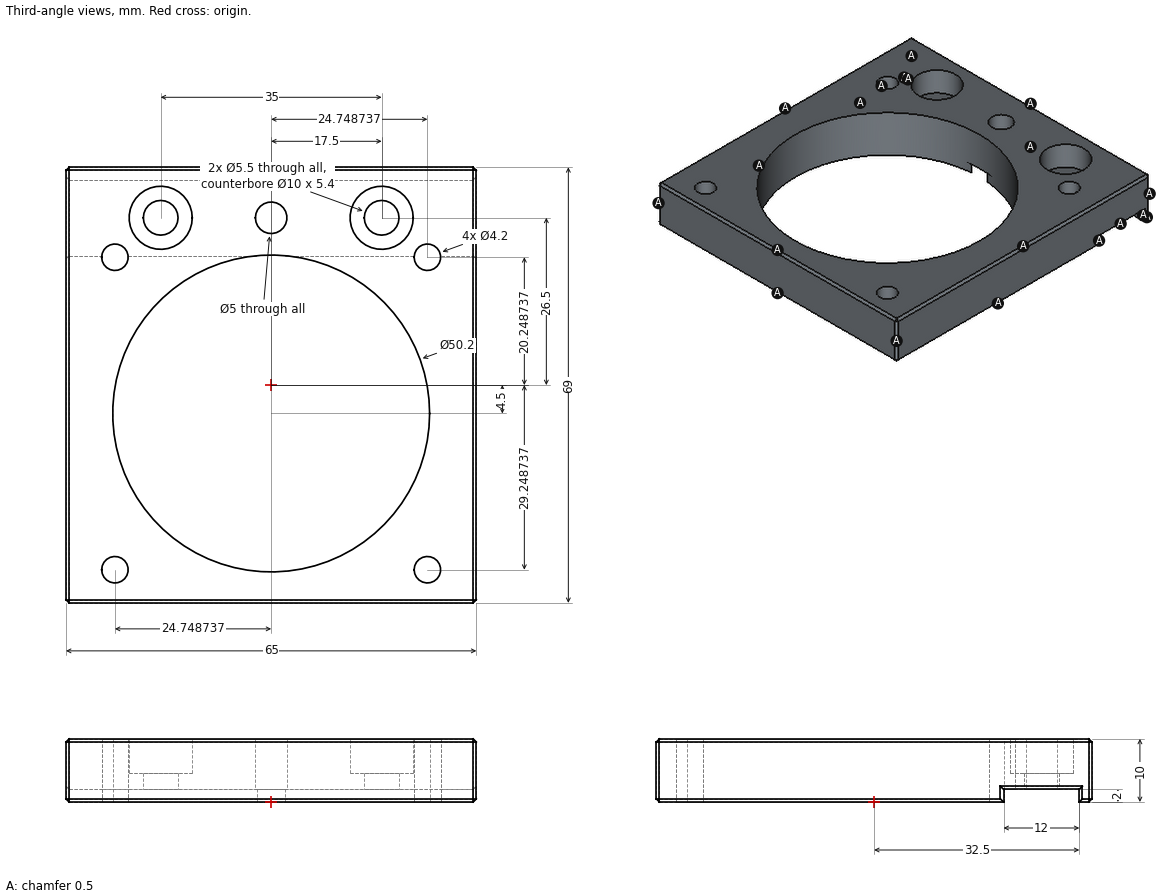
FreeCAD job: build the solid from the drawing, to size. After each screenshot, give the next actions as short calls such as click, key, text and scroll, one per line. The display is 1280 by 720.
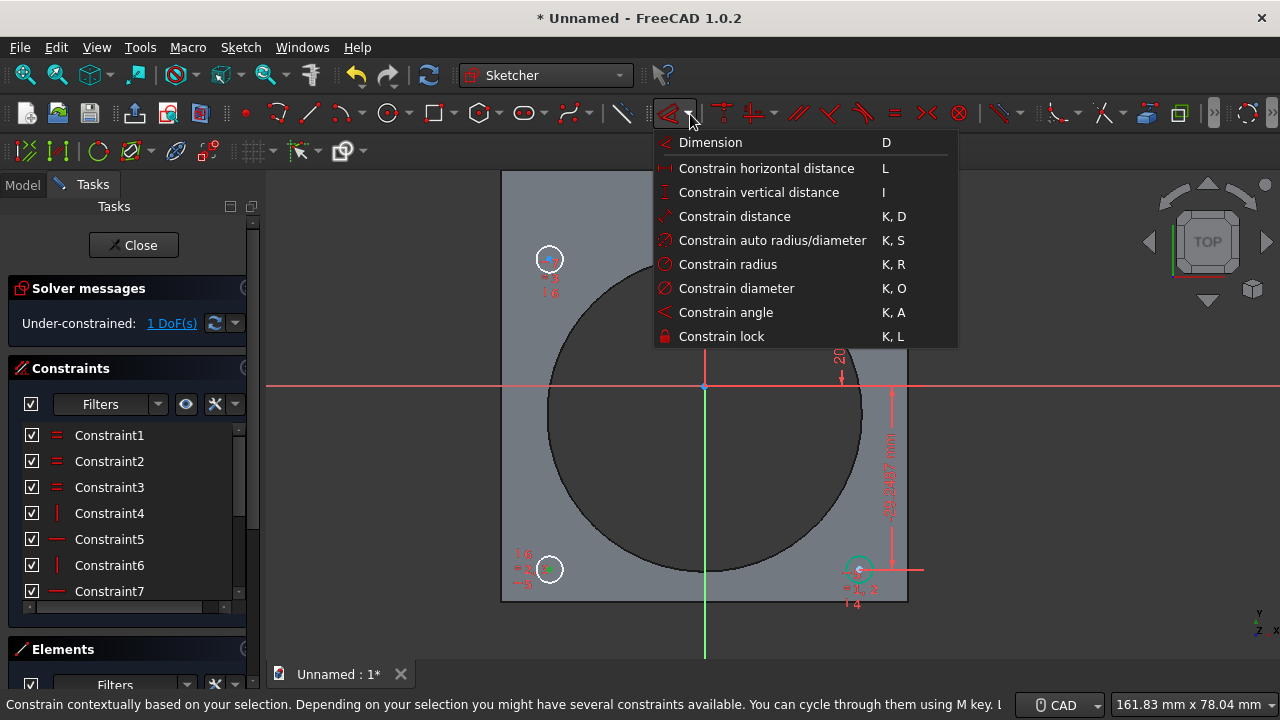
click(806, 168)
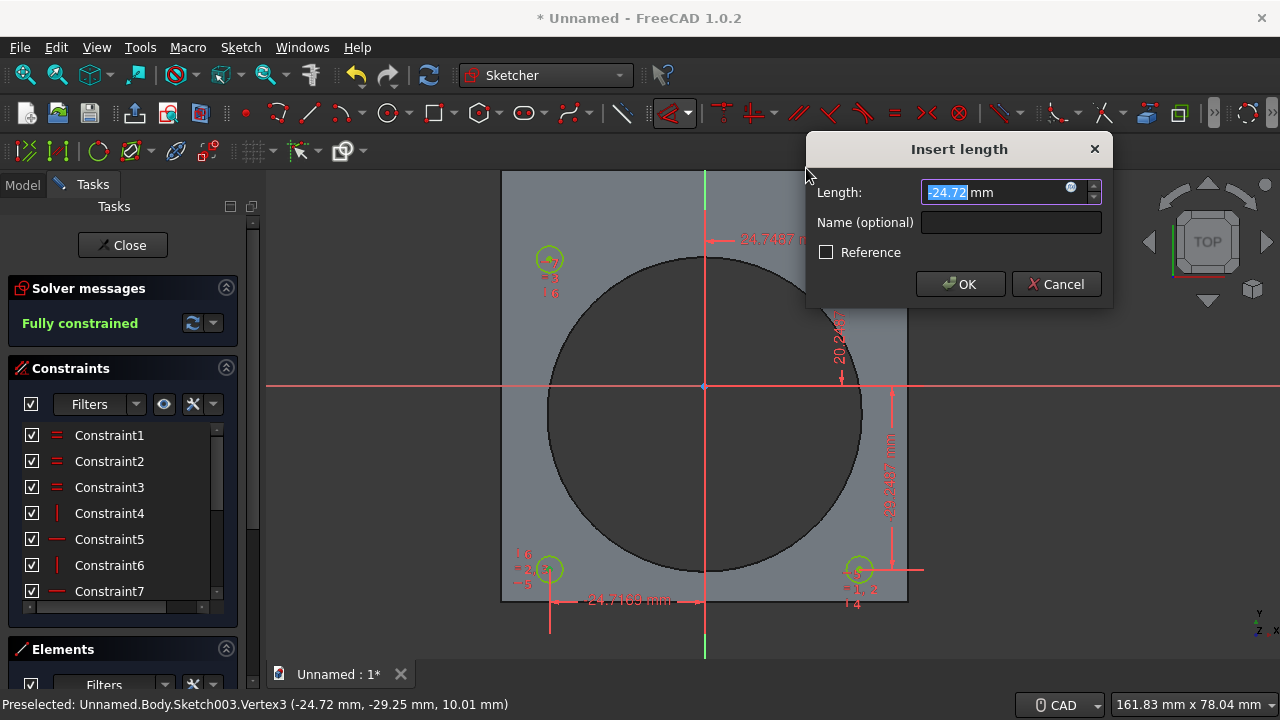
text(-24.748737)
key(Return)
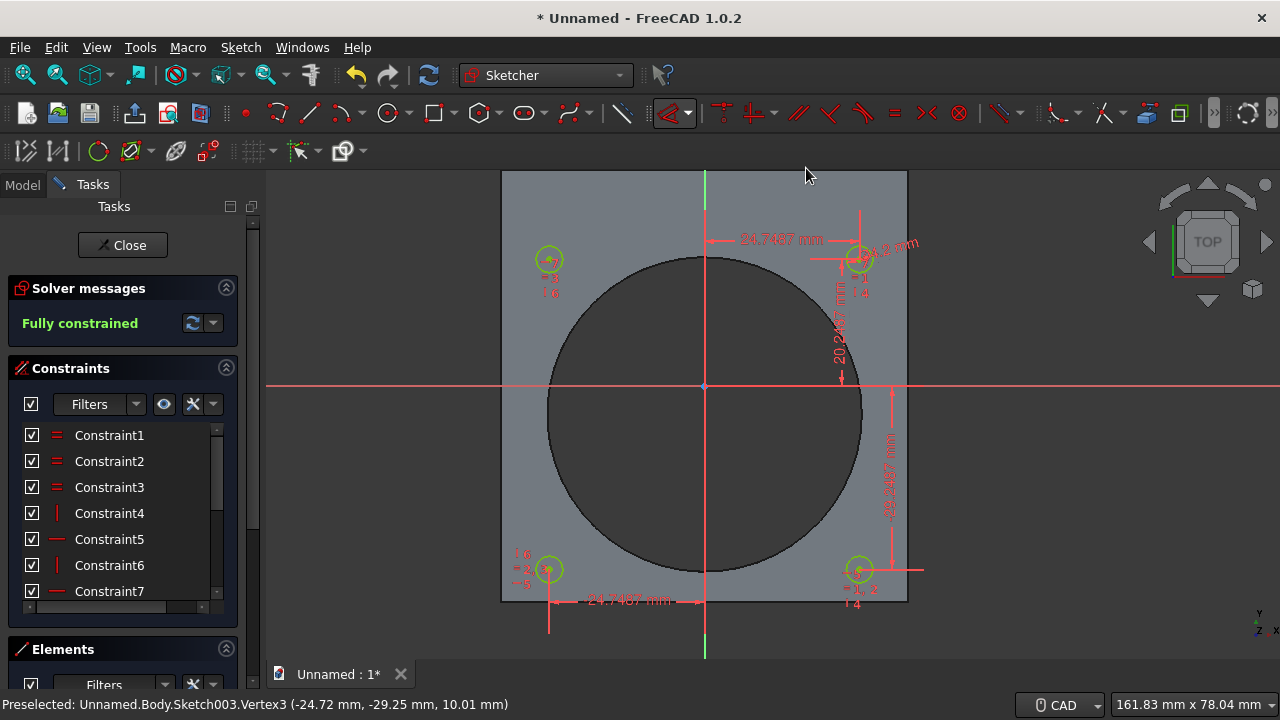
click(123, 245)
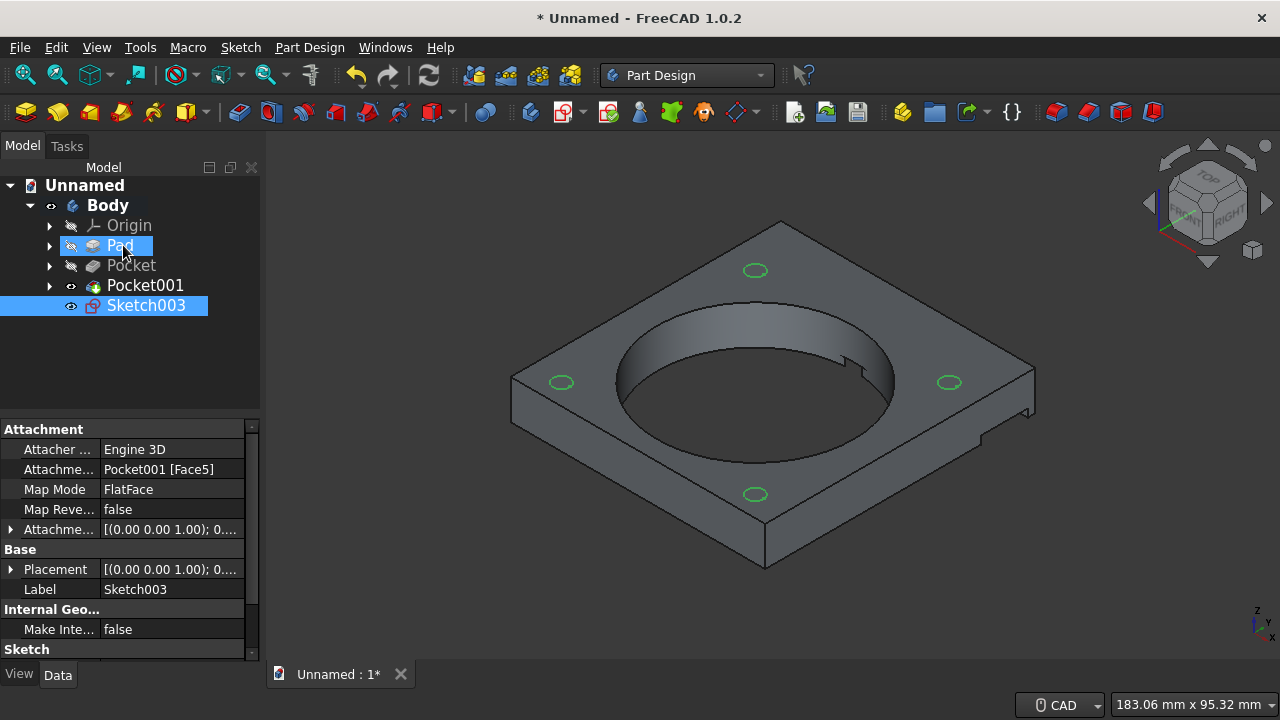
click(240, 112)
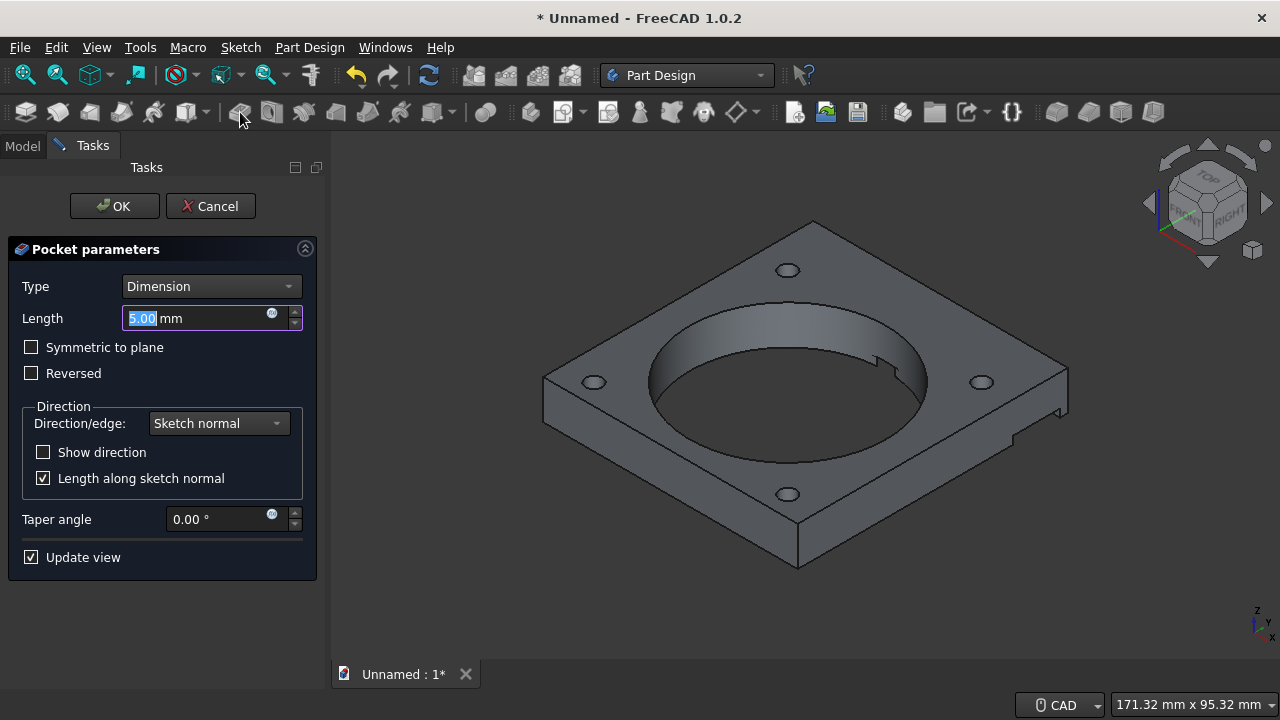
click(212, 286)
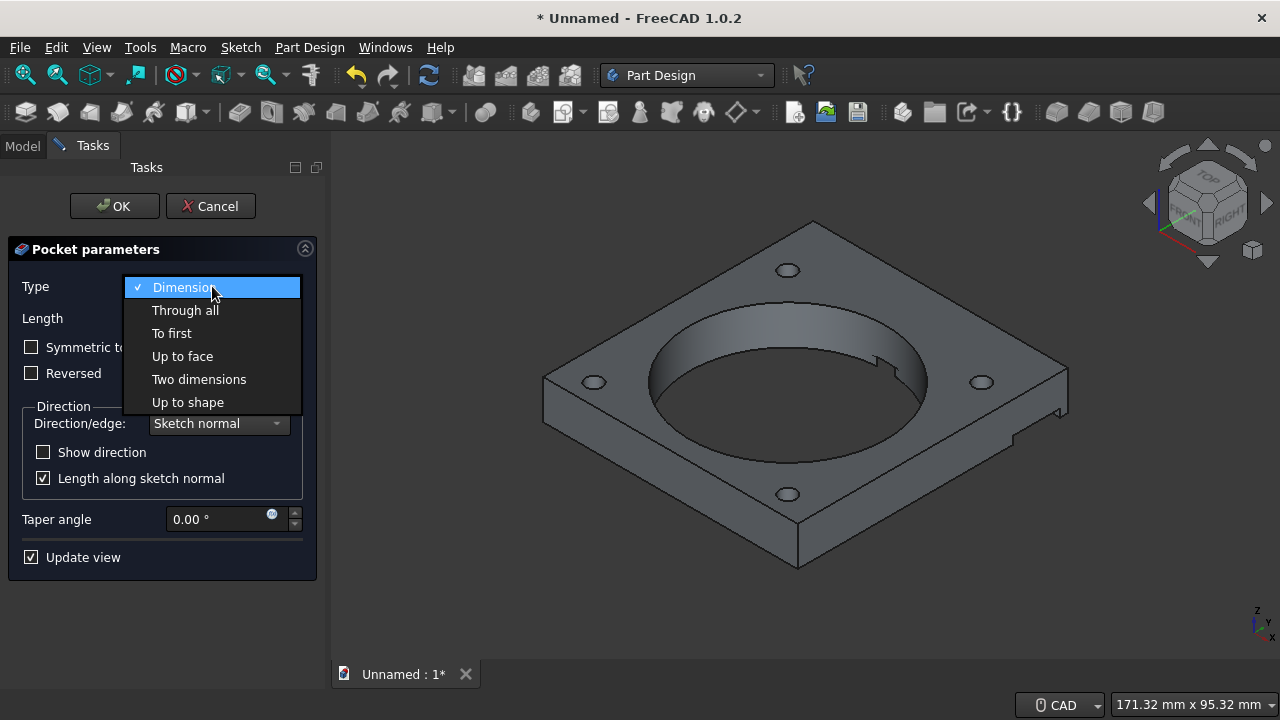
click(212, 310)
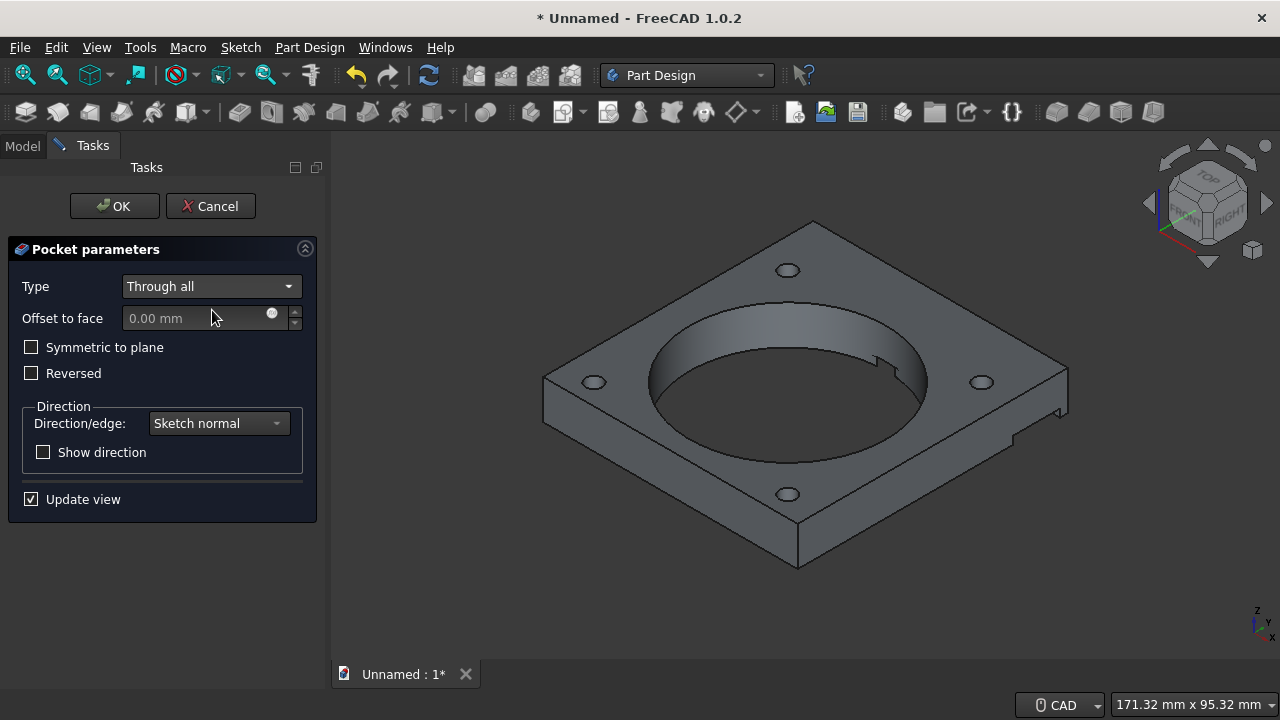
click(115, 206)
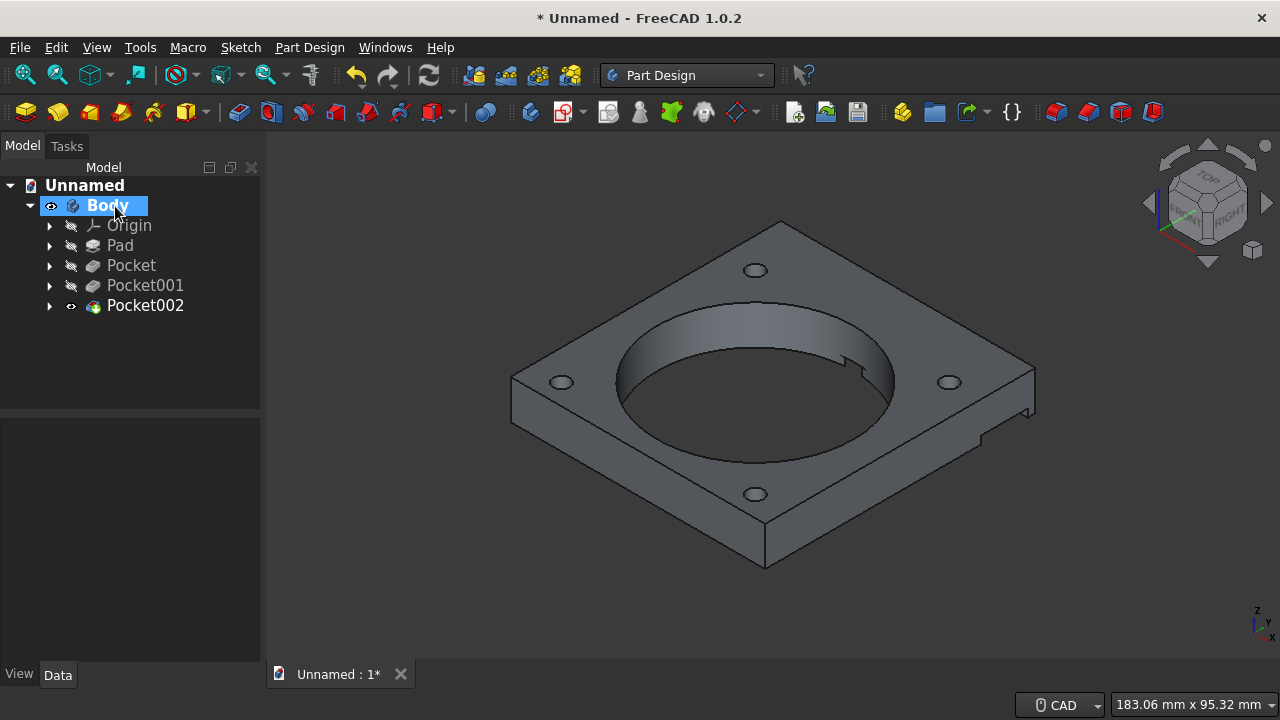
click(962, 347)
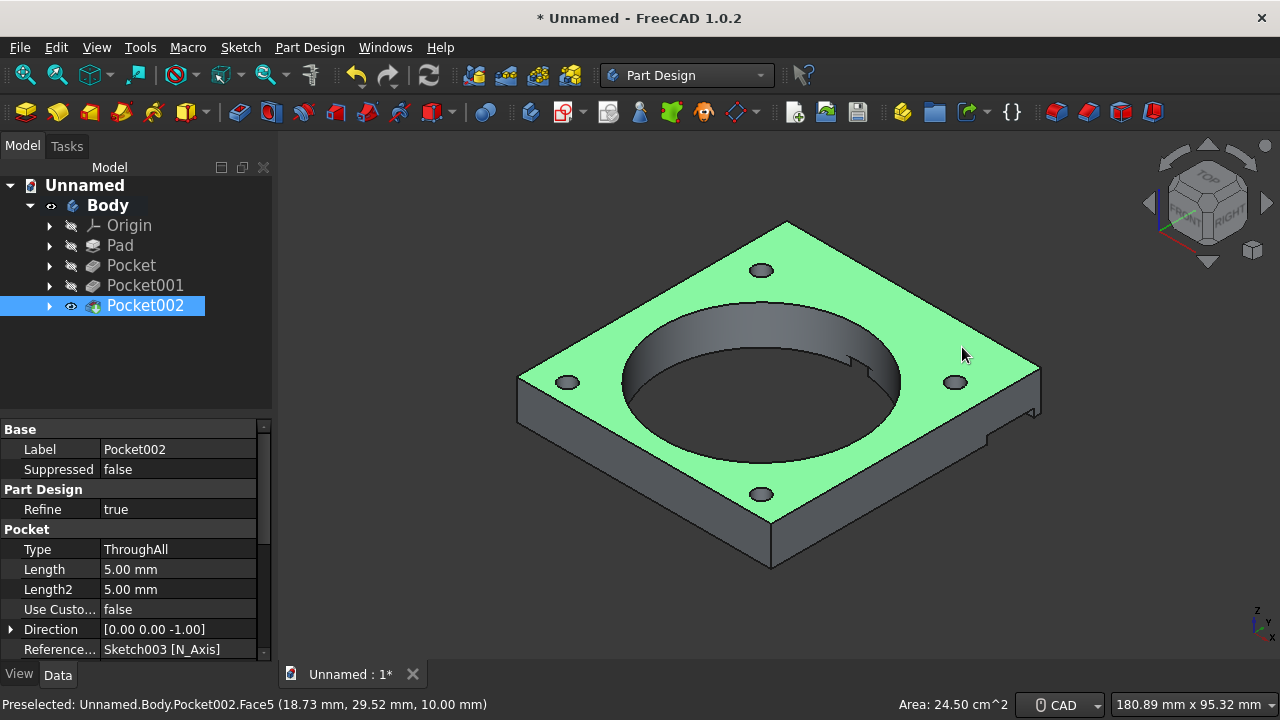
click(564, 112)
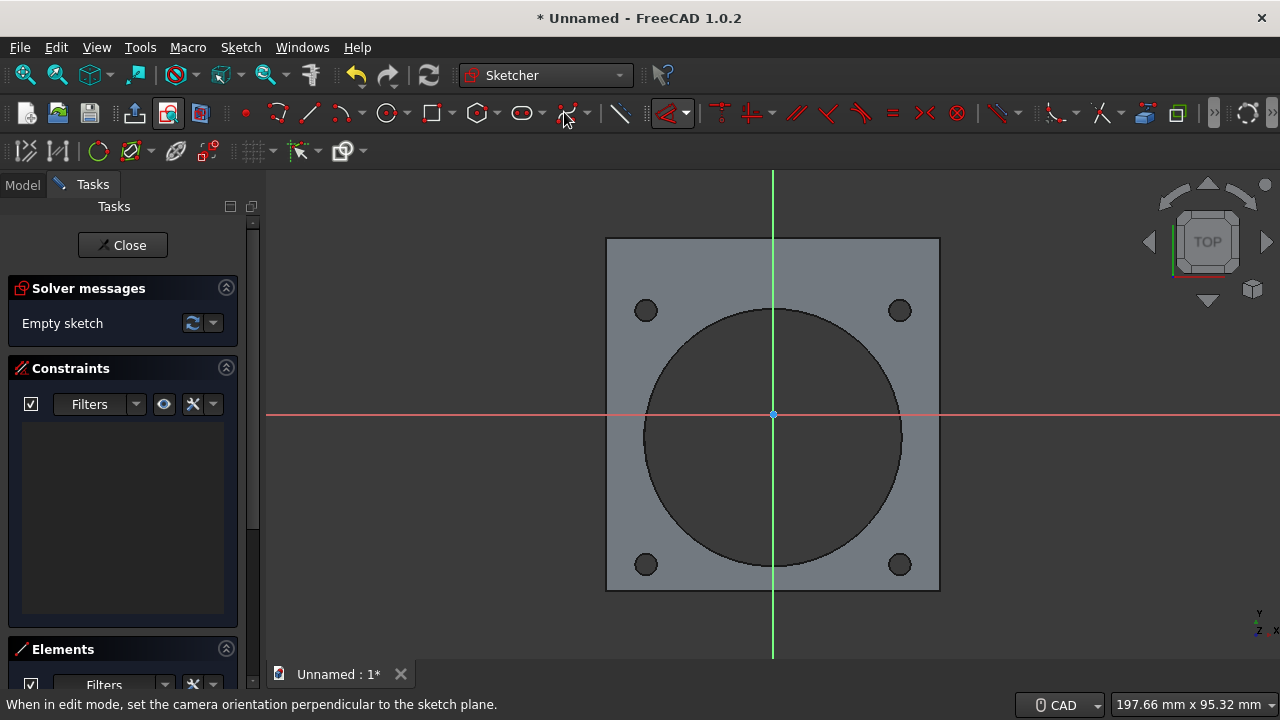
scroll(829, 278, up, 4)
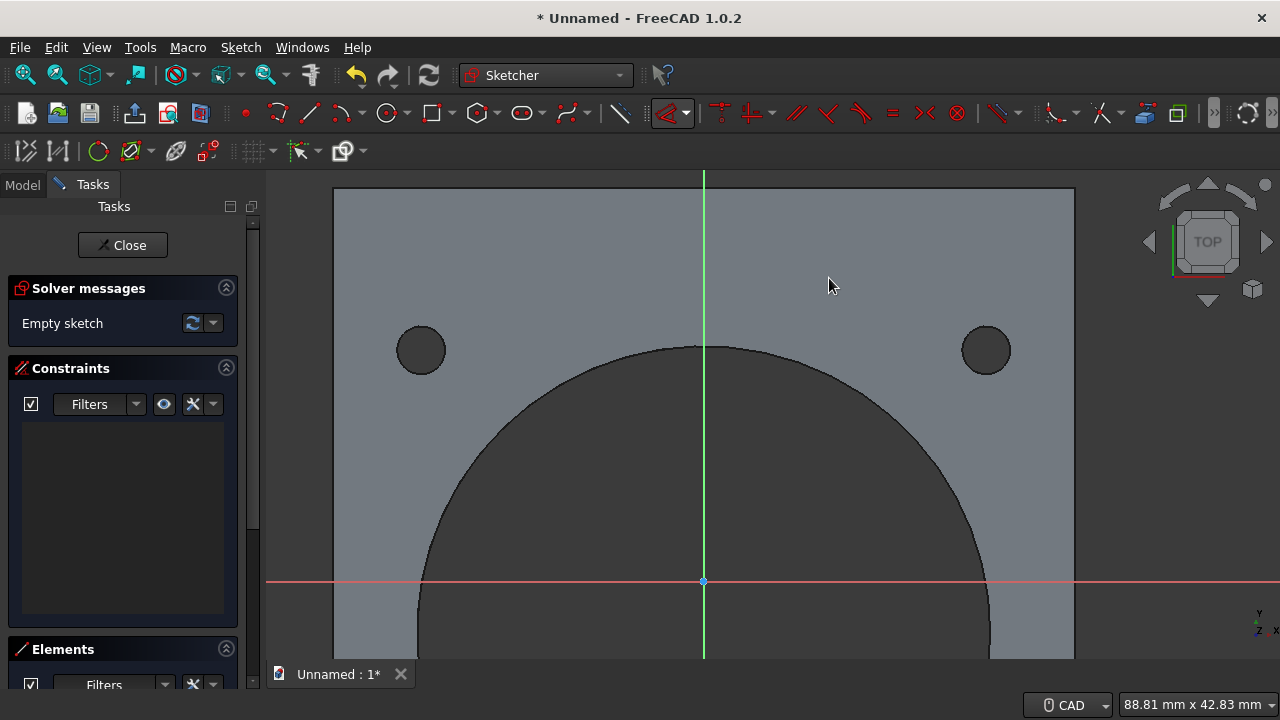
click(388, 114)